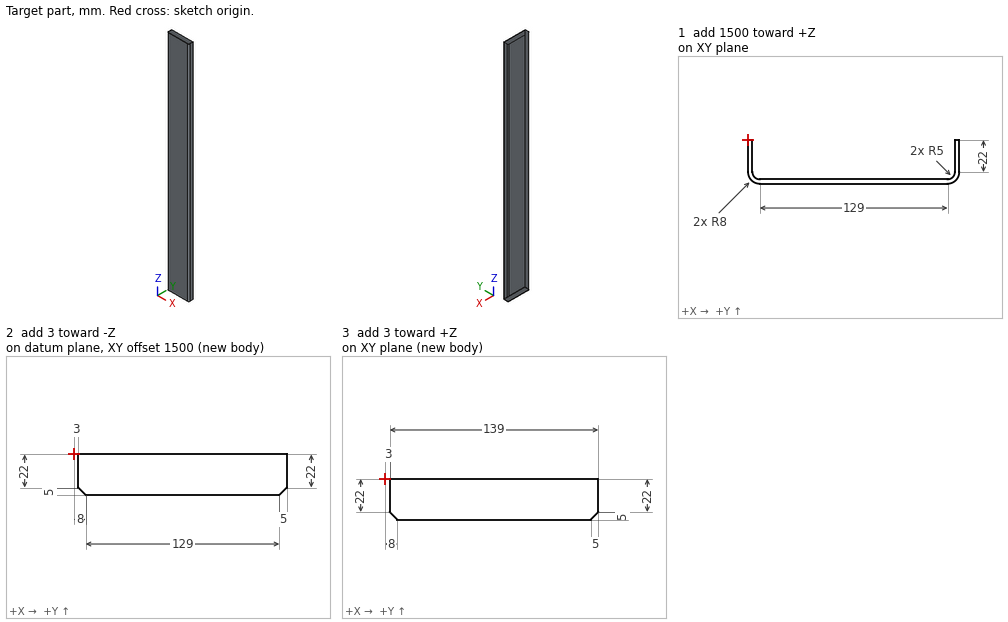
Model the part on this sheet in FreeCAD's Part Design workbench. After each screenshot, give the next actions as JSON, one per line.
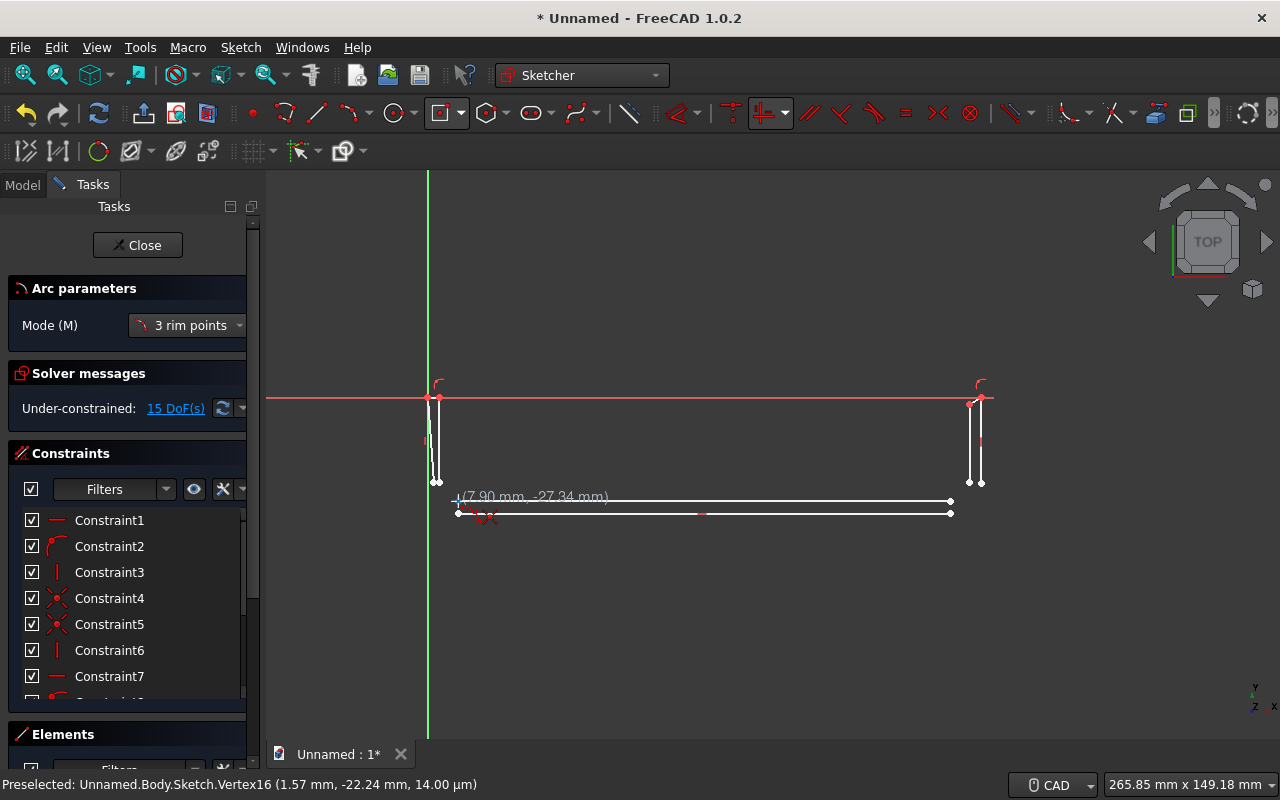
{"action": "scroll", "coordinate": [950, 512], "scroll_direction": "up", "scroll_amount": 2}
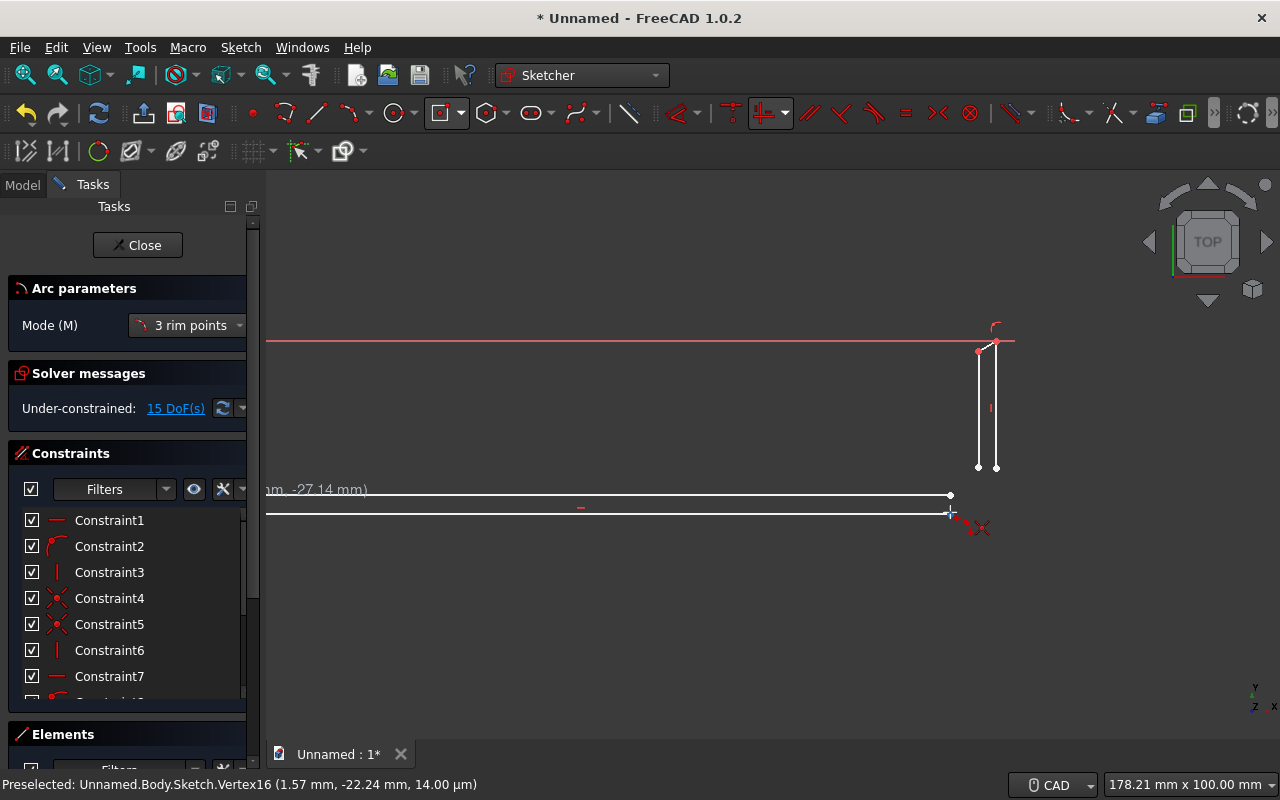
{"action": "left_click", "coordinate": [951, 514]}
{"action": "left_click", "coordinate": [996, 469]}
{"action": "left_click", "coordinate": [983, 498]}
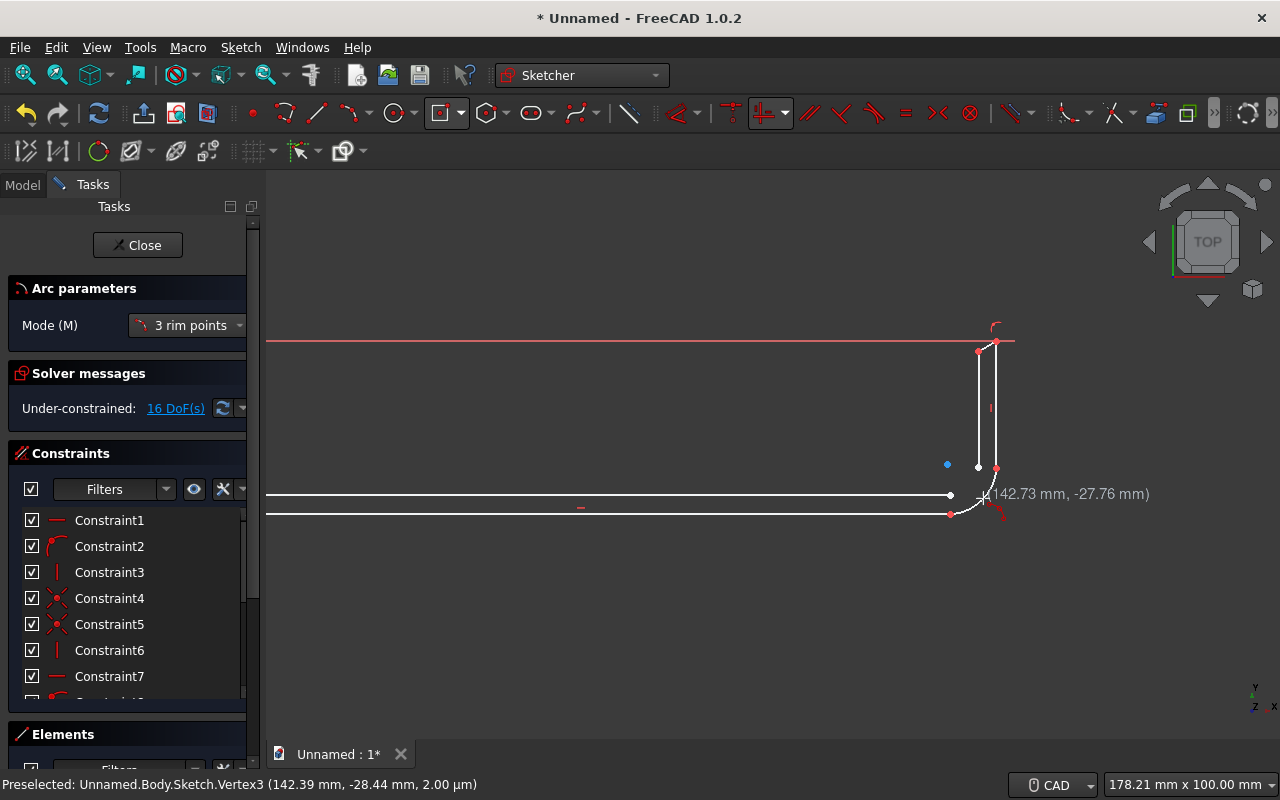
{"action": "left_click", "coordinate": [979, 467]}
{"action": "left_click", "coordinate": [951, 495]}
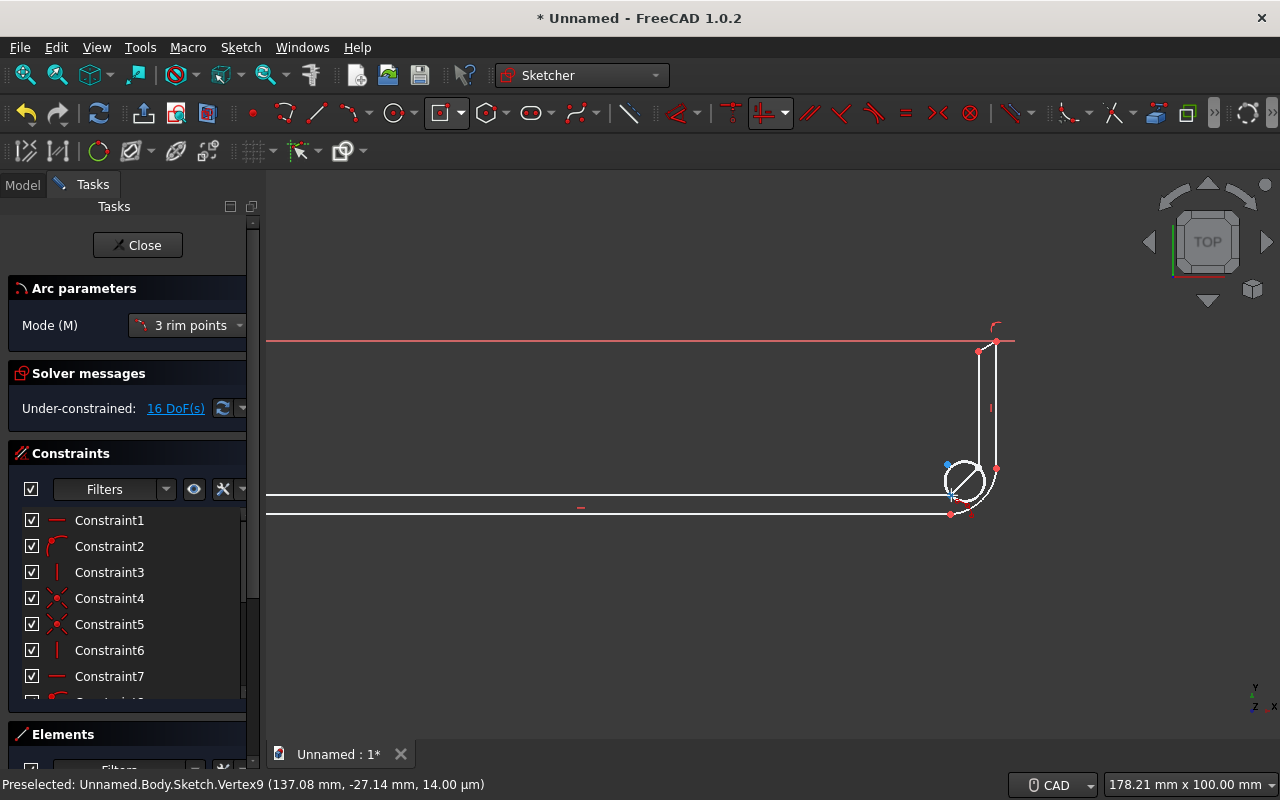
{"action": "scroll", "coordinate": [970, 486], "scroll_direction": "up", "scroll_amount": 4}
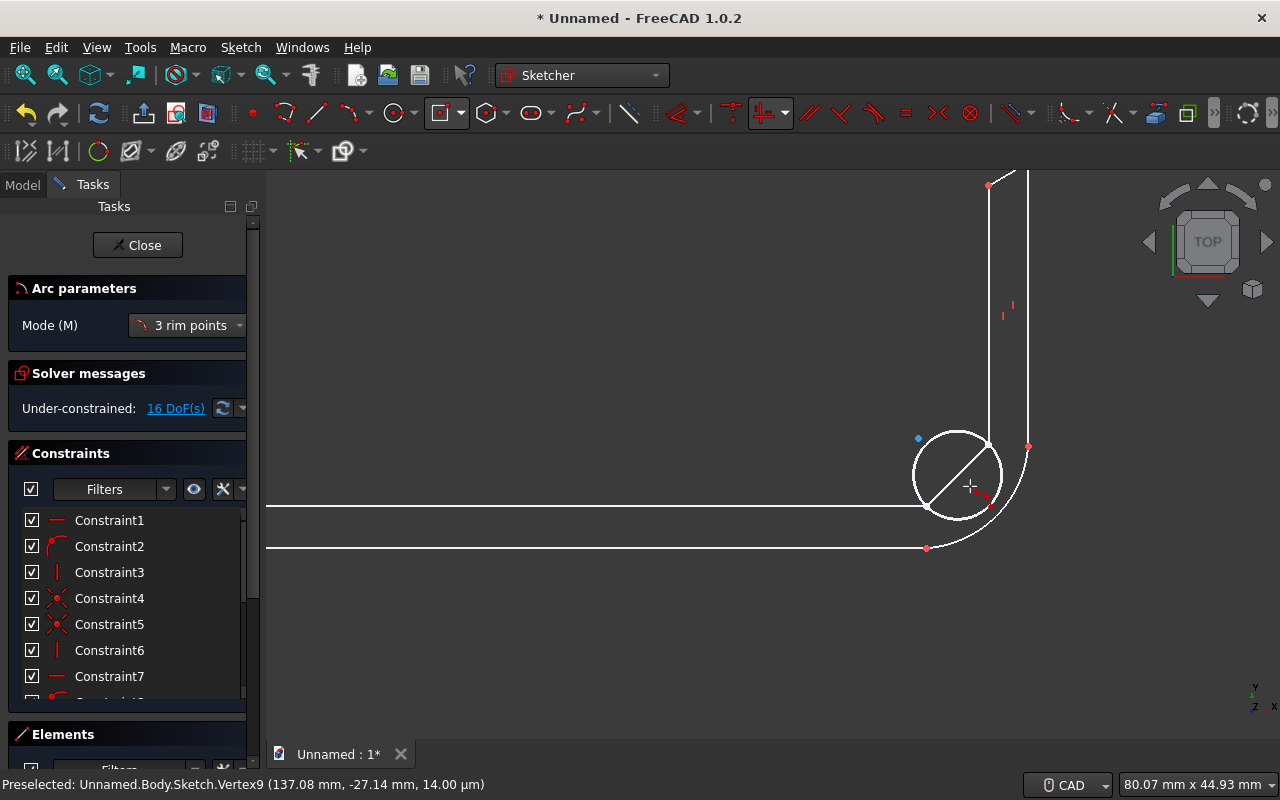
{"action": "left_click", "coordinate": [970, 486]}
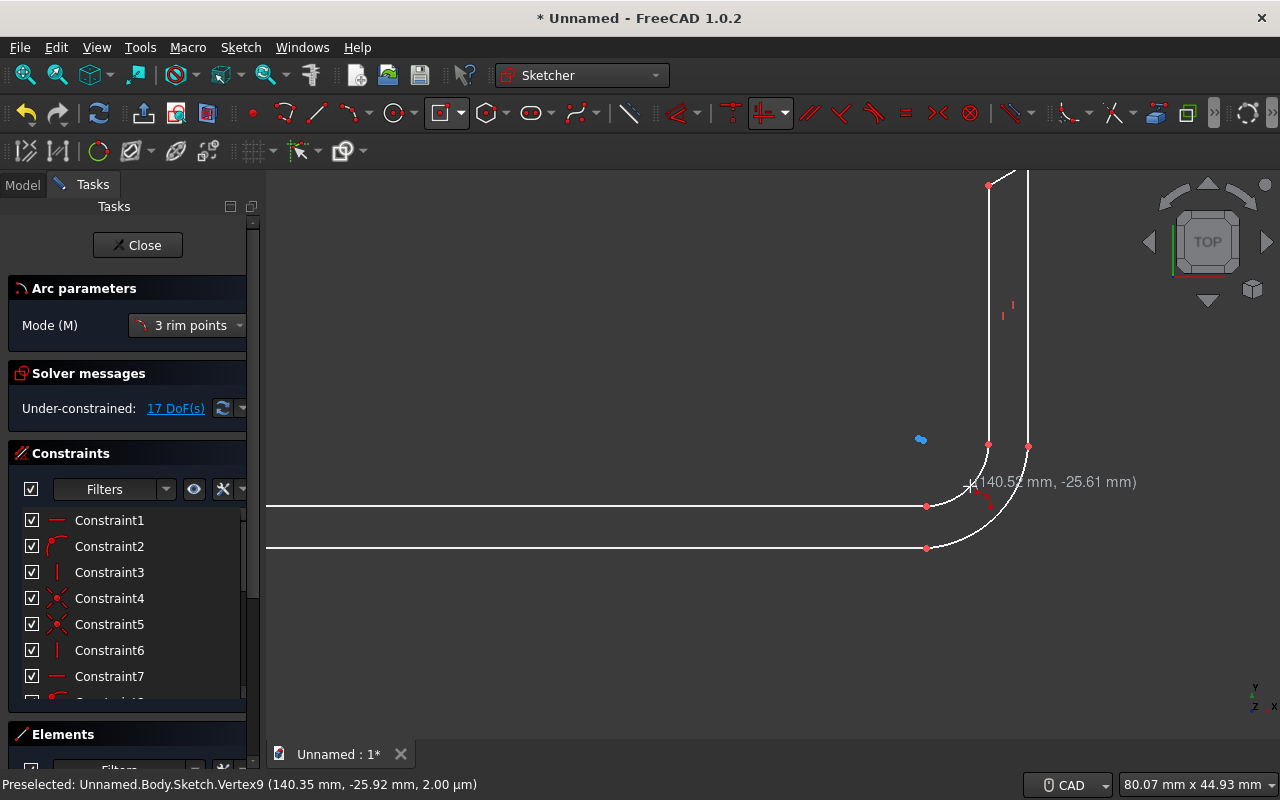
{"action": "scroll", "coordinate": [961, 498], "scroll_direction": "down", "scroll_amount": 6}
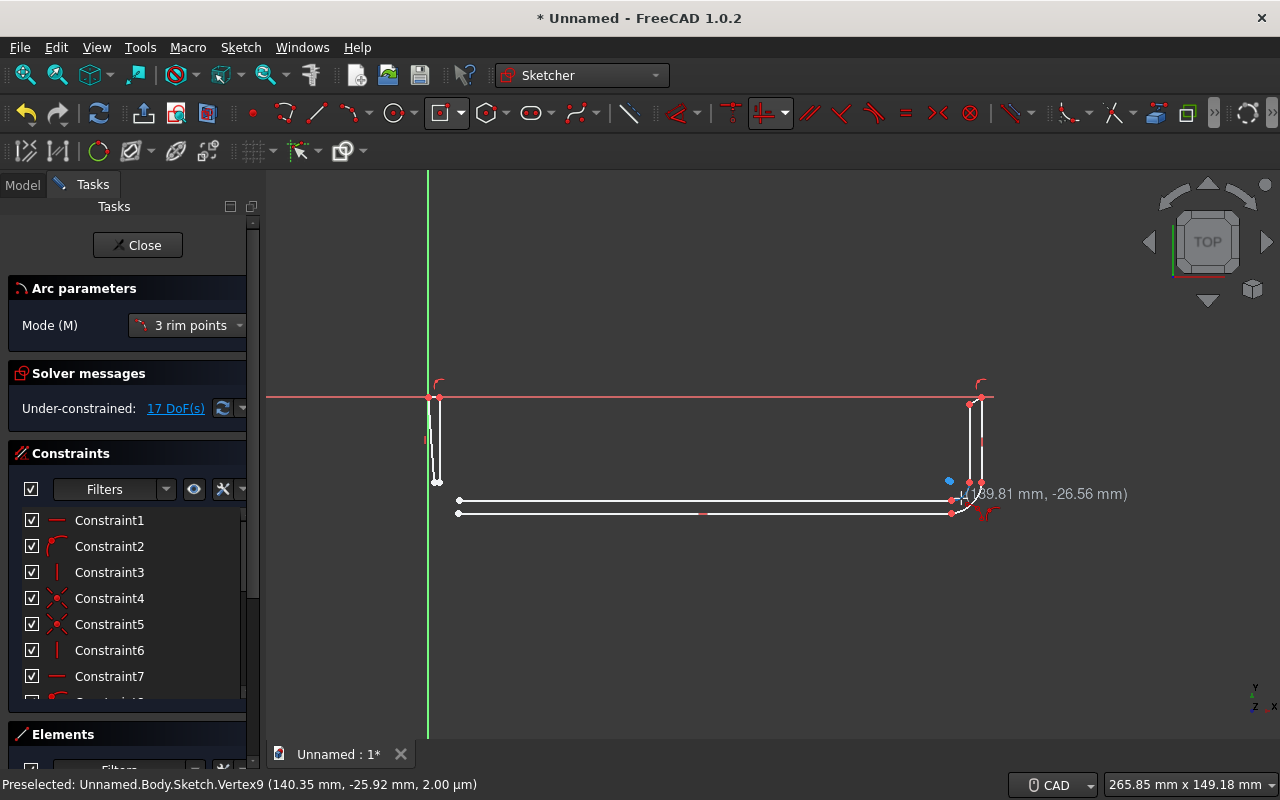
{"action": "scroll", "coordinate": [459, 500], "scroll_direction": "up", "scroll_amount": 2}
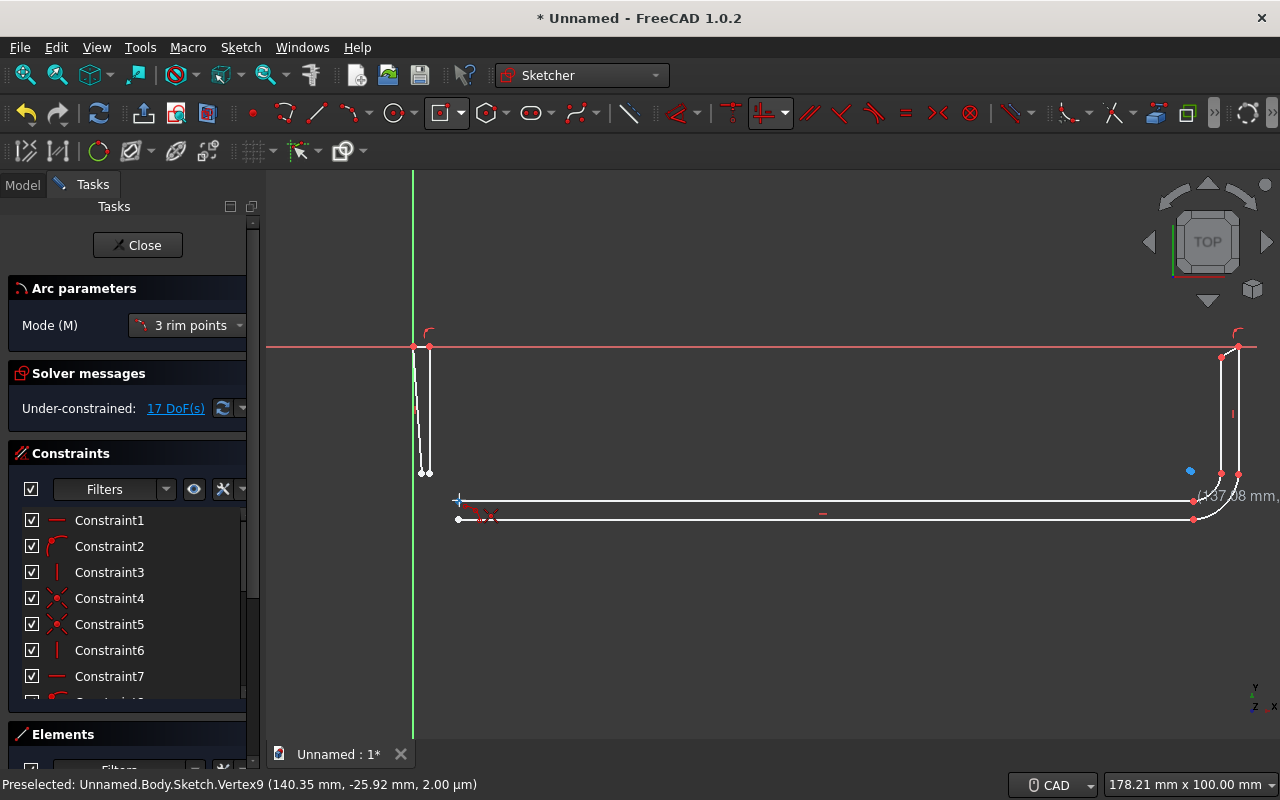
{"action": "left_click", "coordinate": [459, 501]}
{"action": "left_click", "coordinate": [430, 473]}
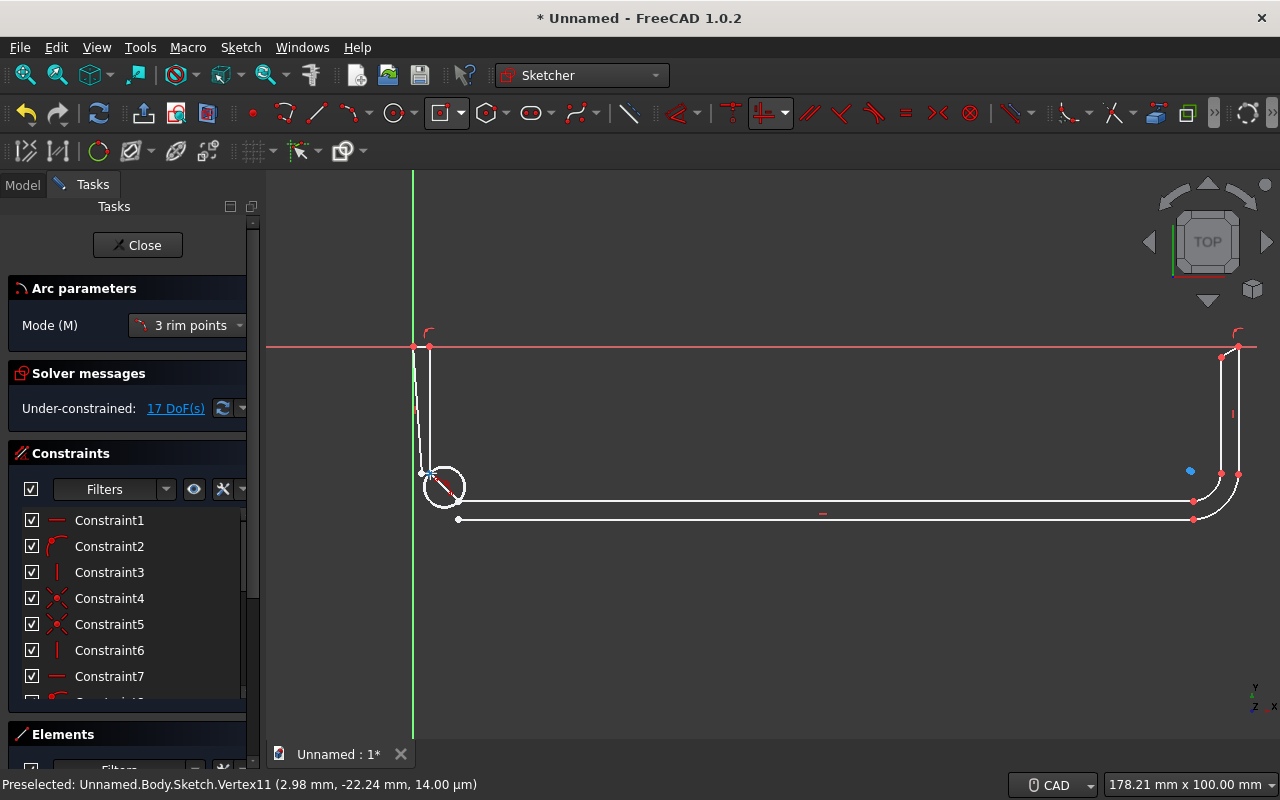
{"action": "scroll", "coordinate": [438, 492], "scroll_direction": "up", "scroll_amount": 4}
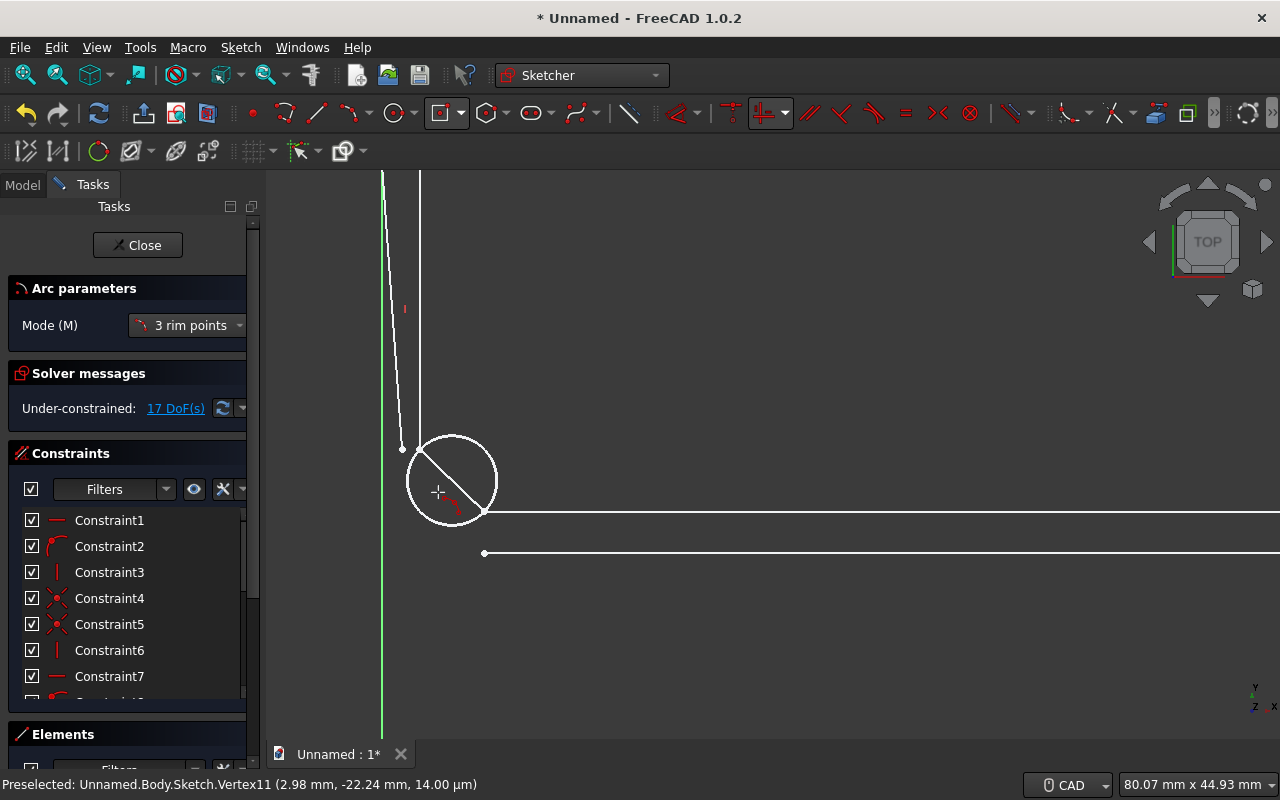
{"action": "left_click", "coordinate": [439, 491]}